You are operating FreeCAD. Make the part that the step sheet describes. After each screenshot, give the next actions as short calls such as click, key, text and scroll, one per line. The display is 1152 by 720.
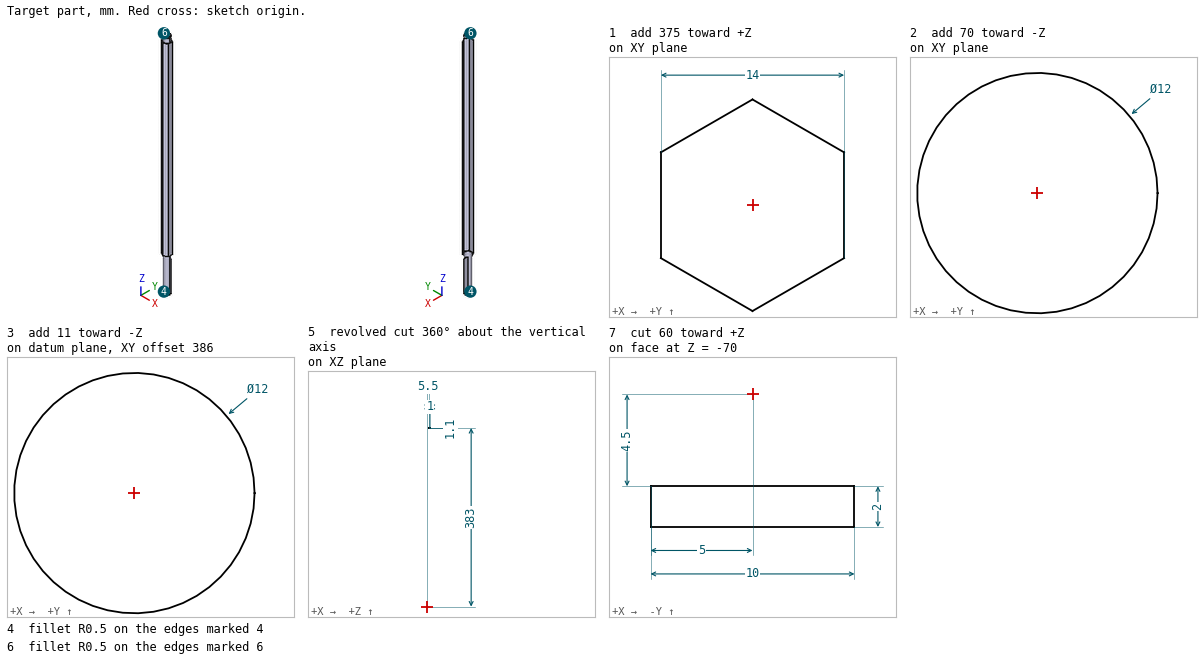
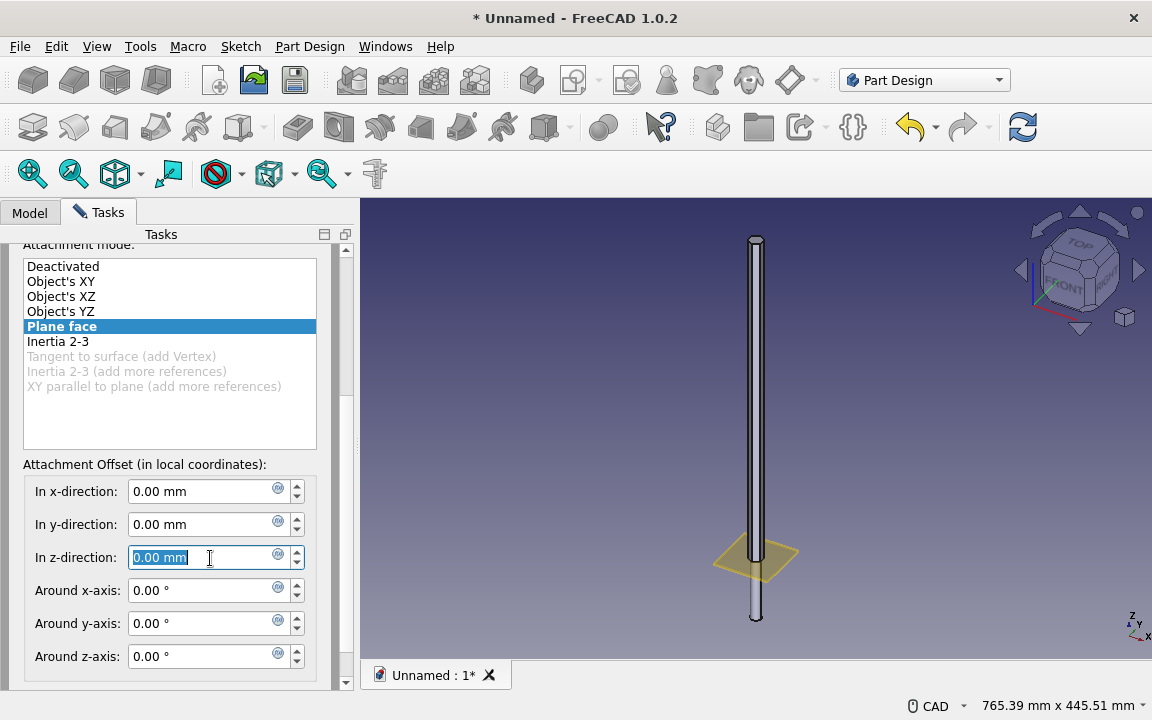
text(386)
key(Tab)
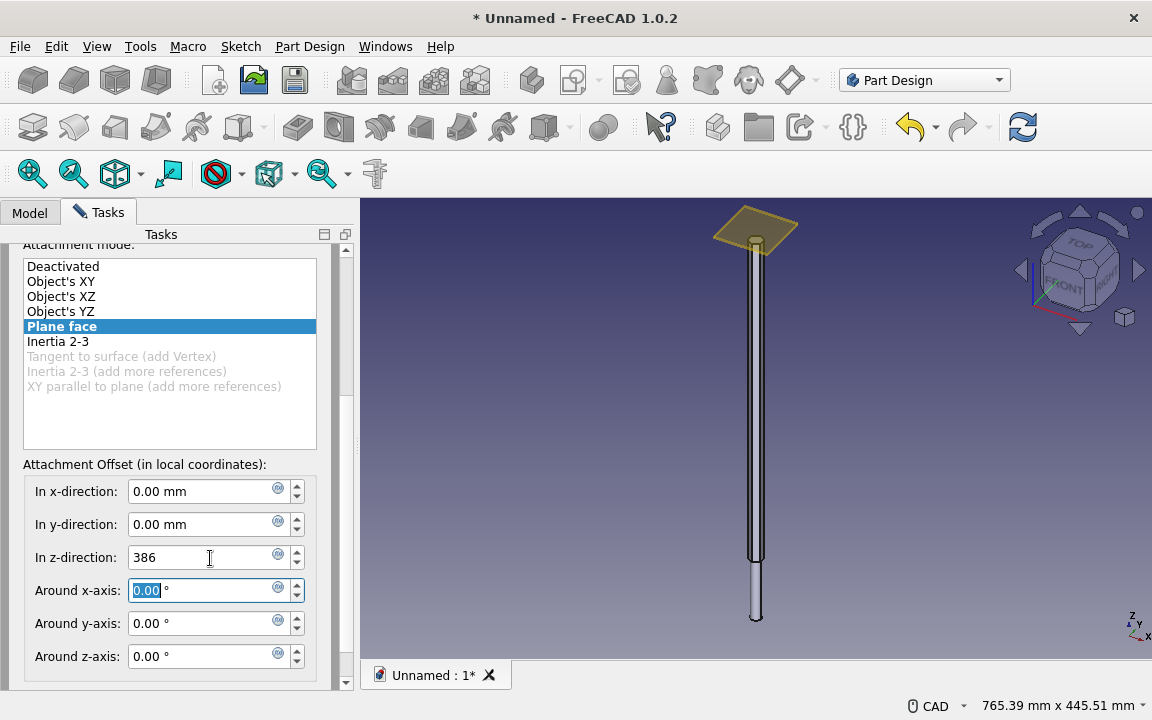
scroll(346, 467, up, 5)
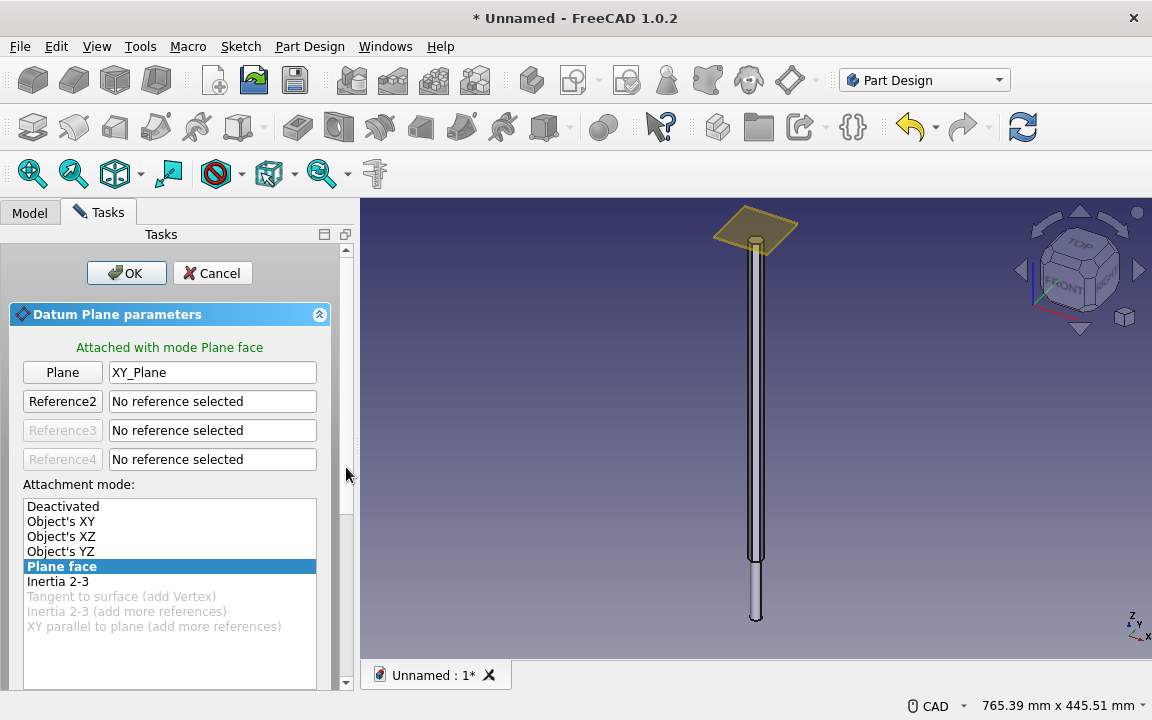
click(127, 273)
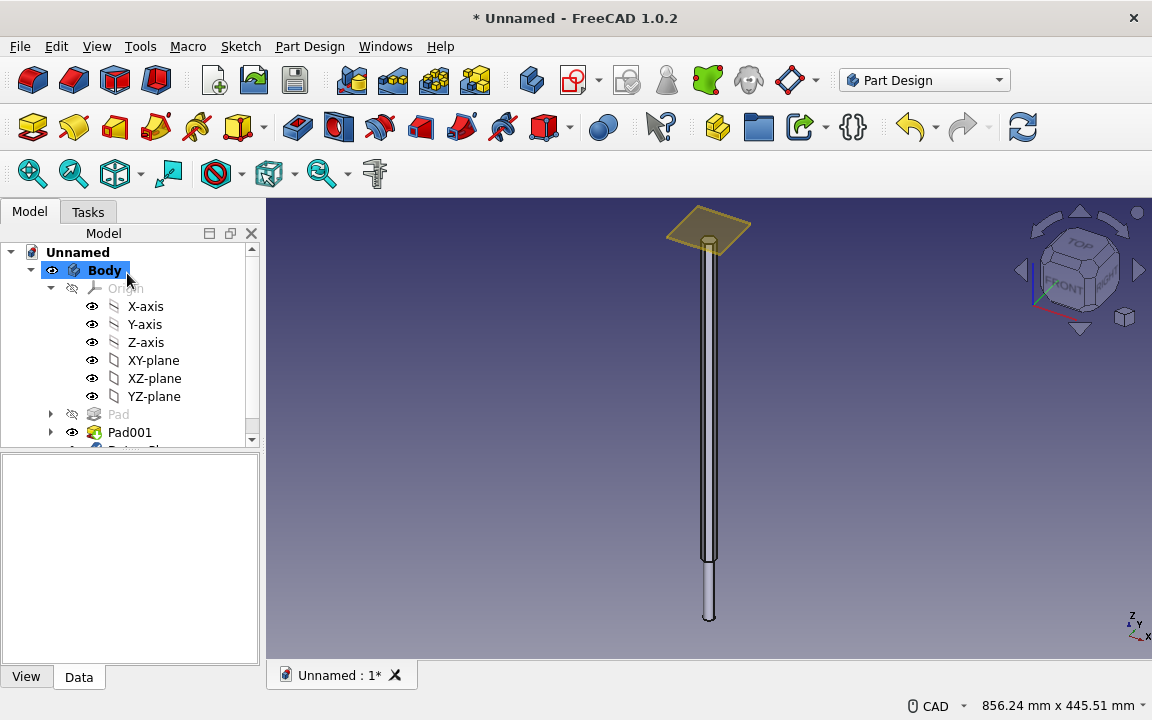
scroll(101, 338, down, 3)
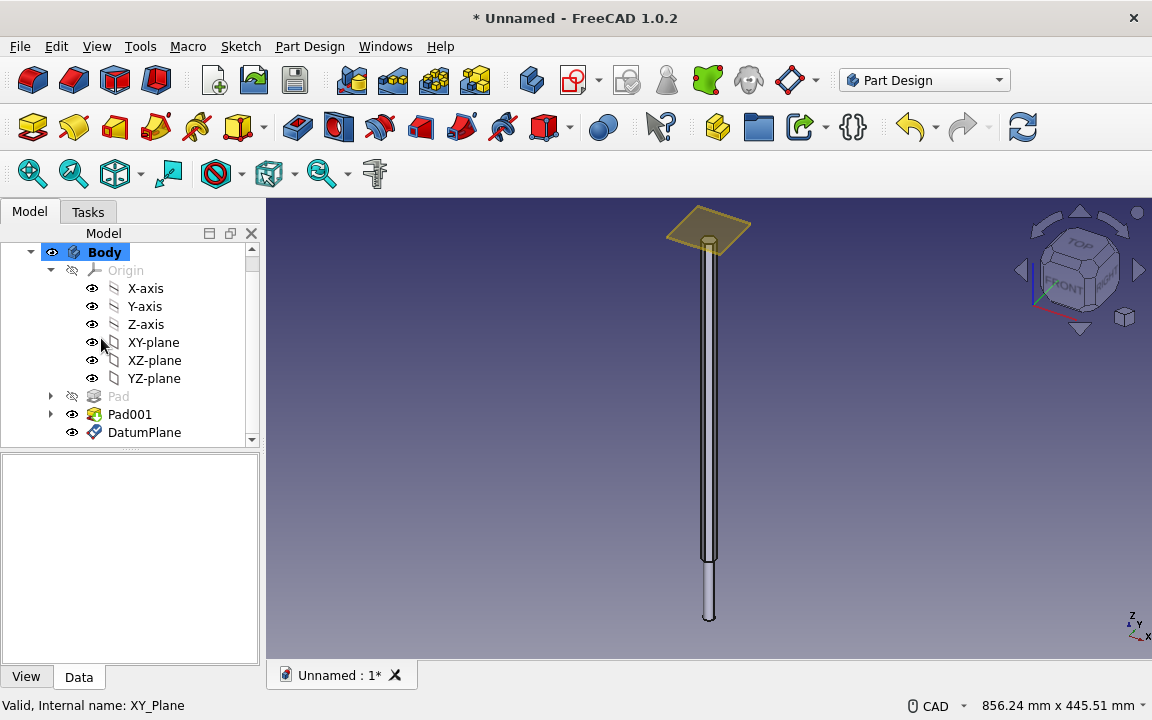
click(117, 432)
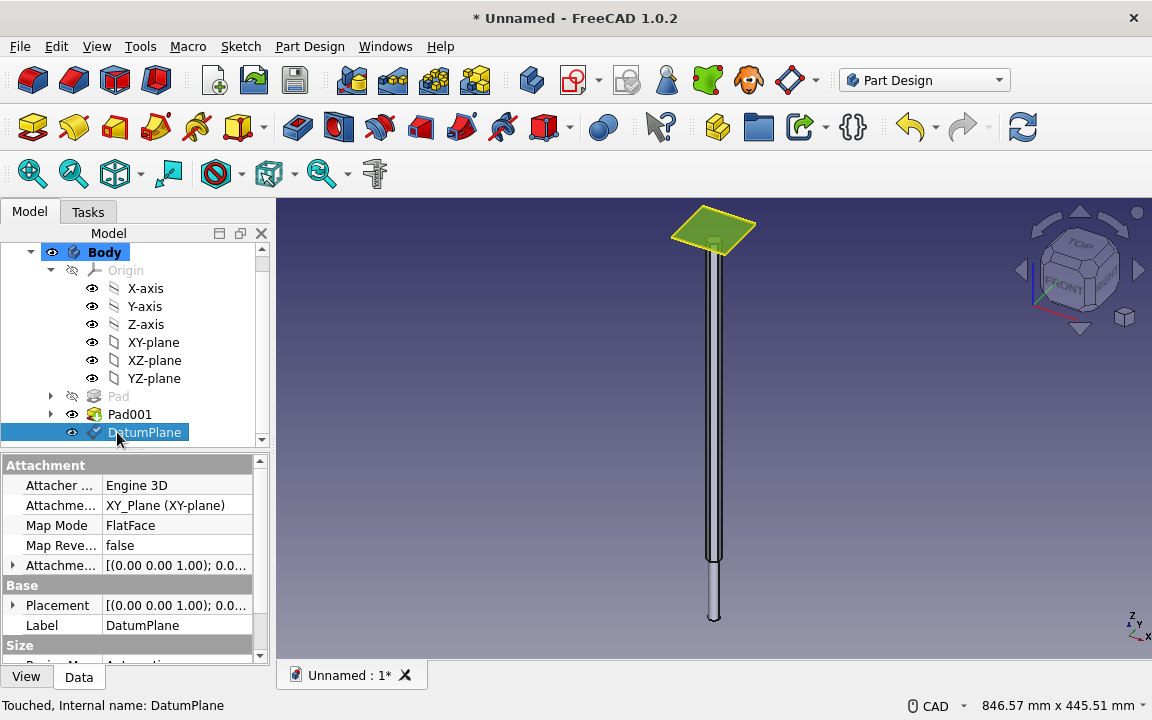
click(572, 80)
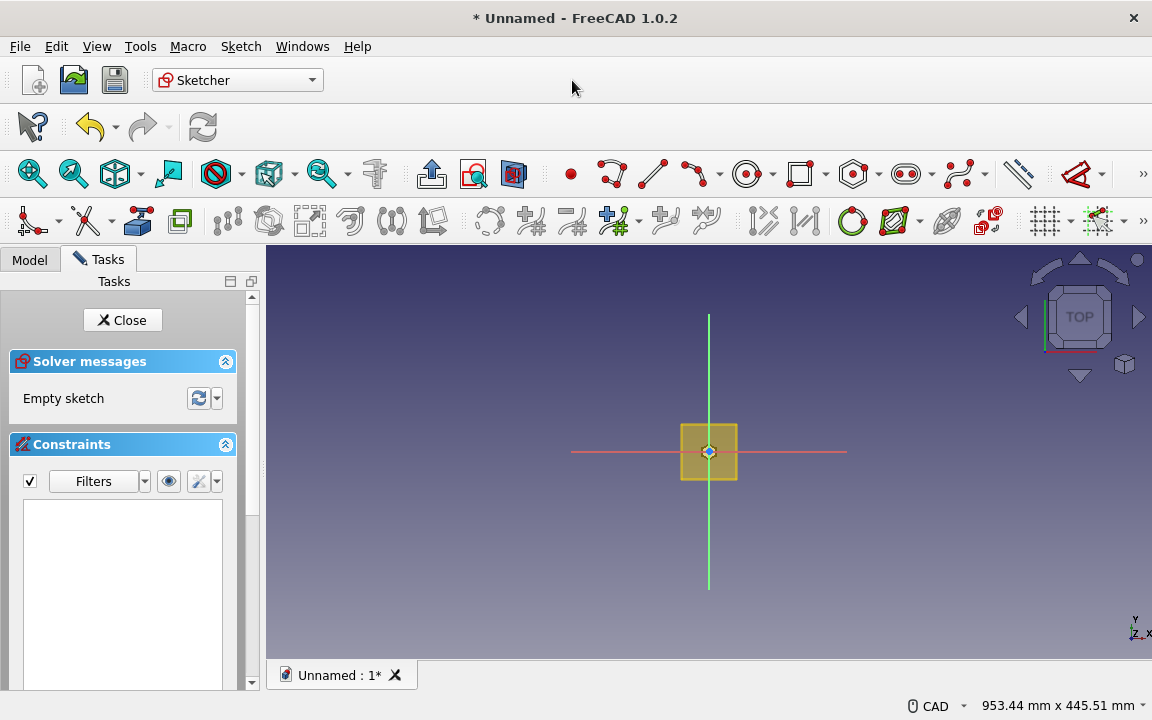
scroll(713, 452, up, 15)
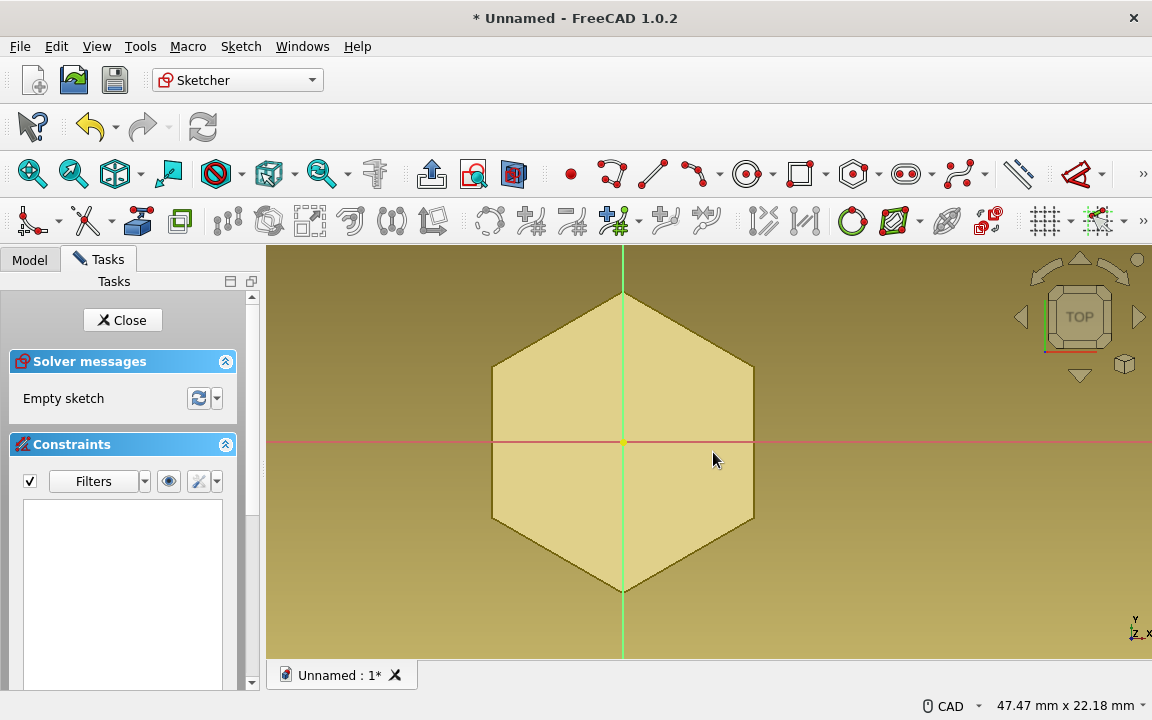
click(746, 174)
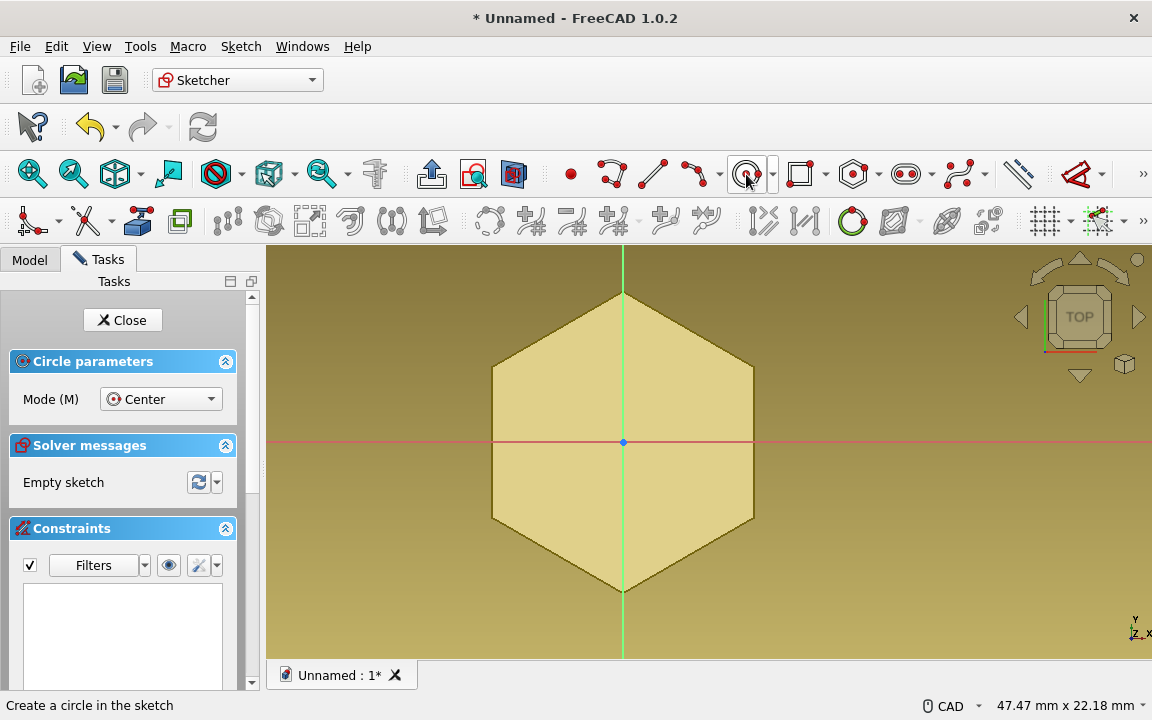
click(623, 442)
move(702, 363)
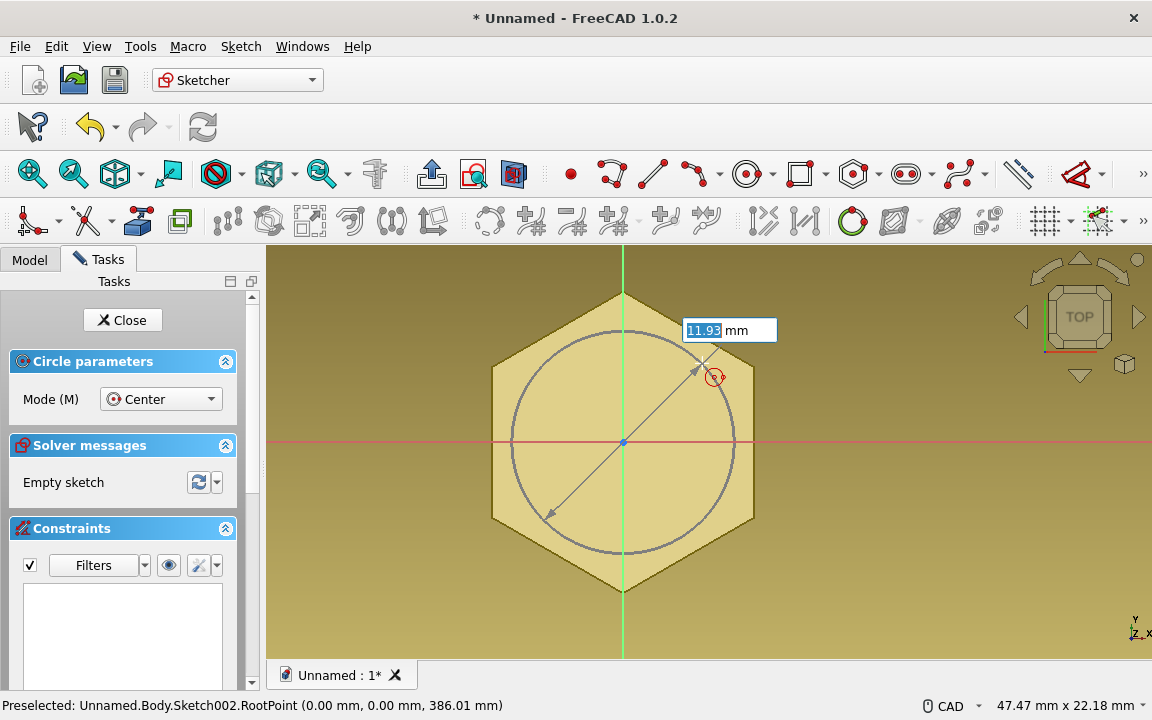
text(12)
key(Return)
key(Escape)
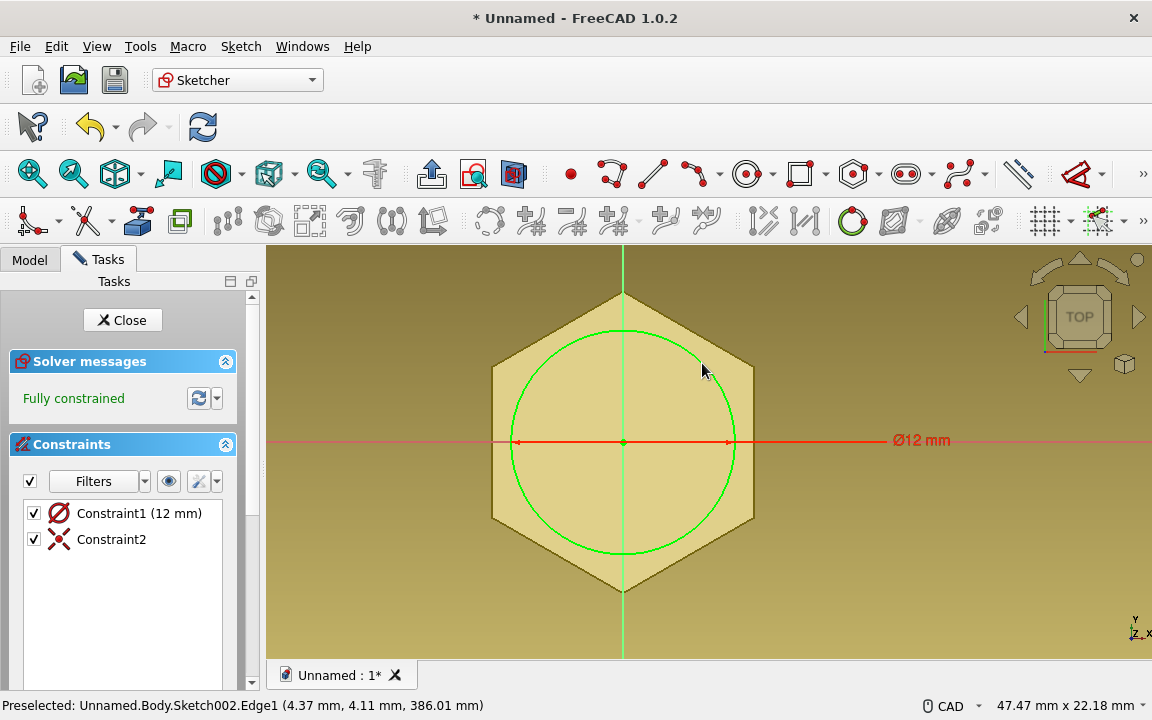
click(123, 320)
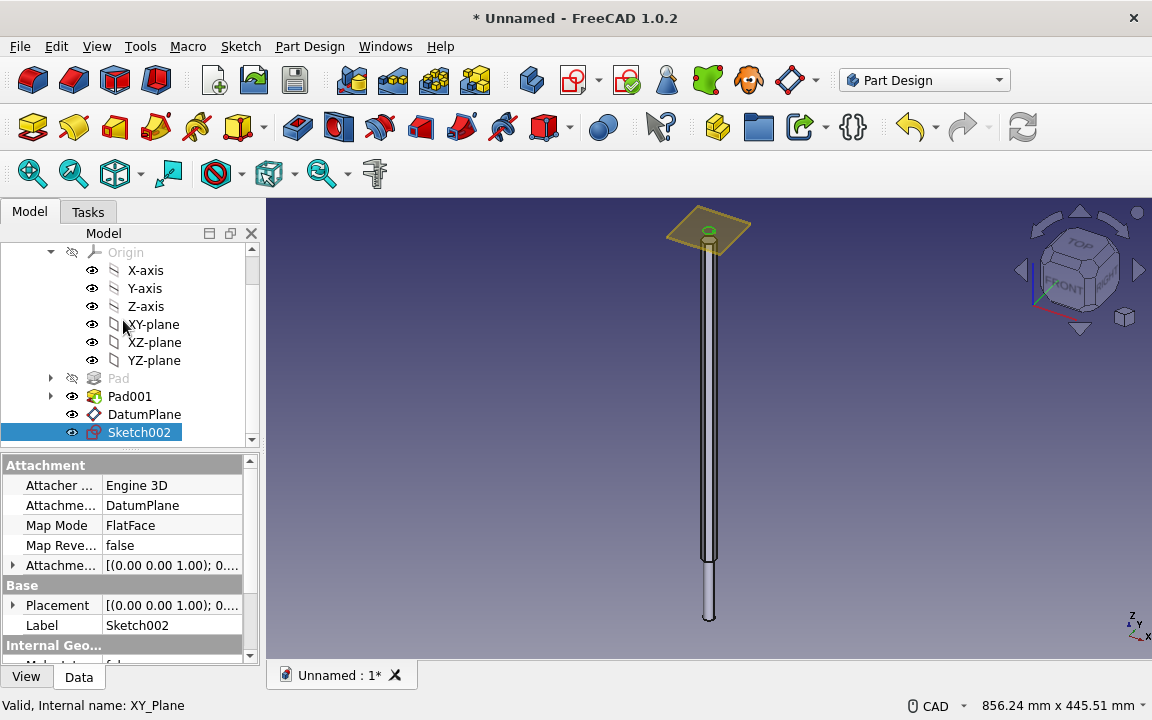
click(33, 128)